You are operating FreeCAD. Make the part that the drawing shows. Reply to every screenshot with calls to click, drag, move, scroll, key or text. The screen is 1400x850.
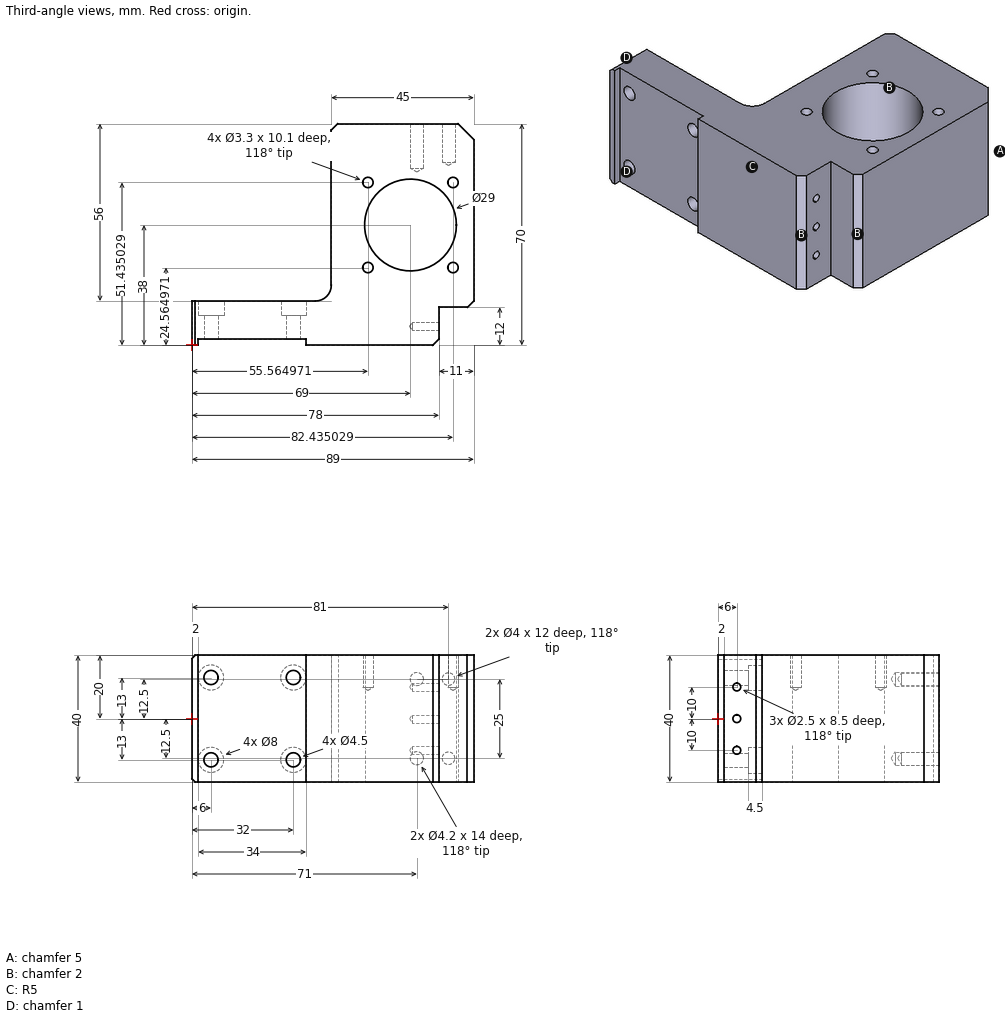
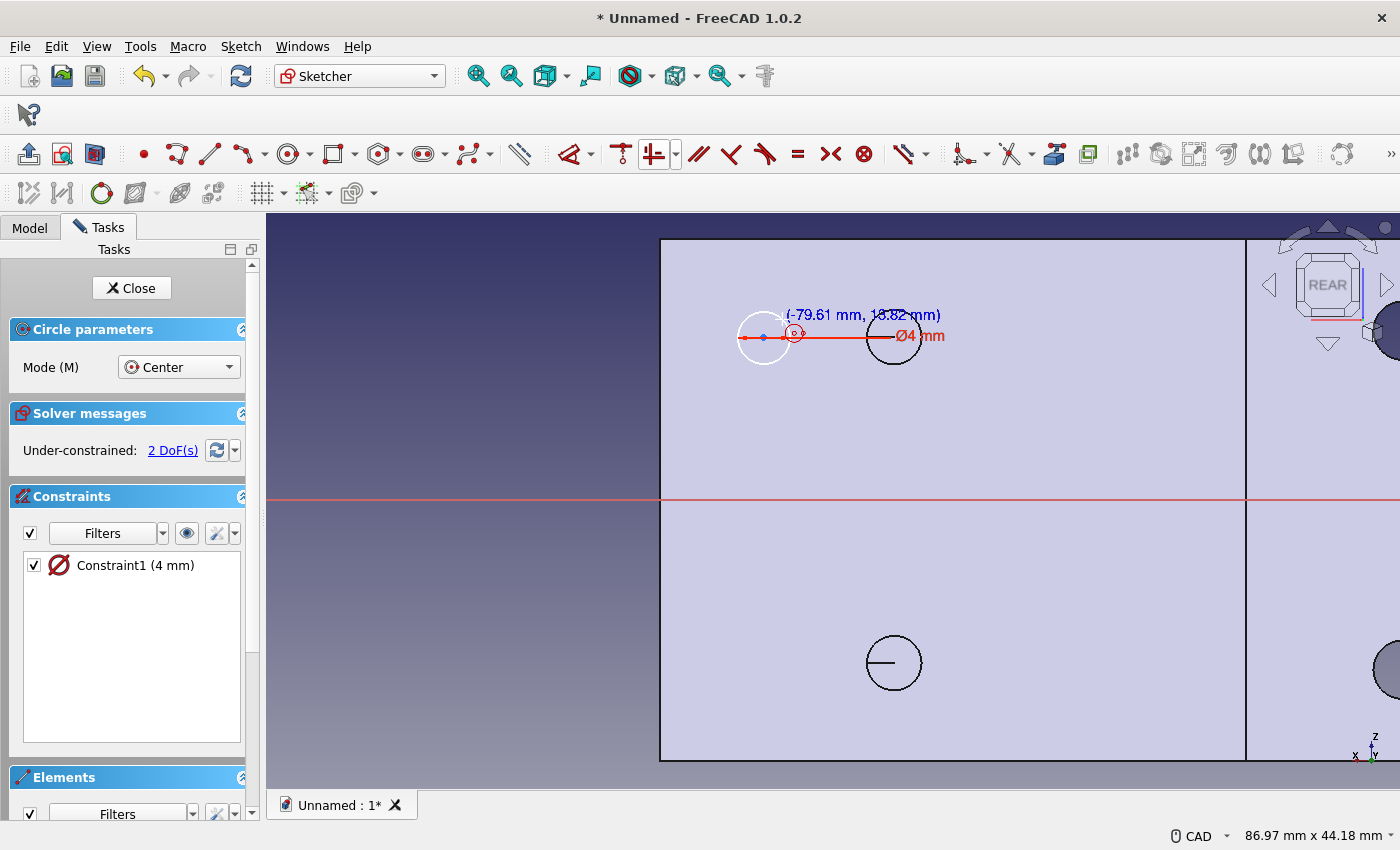
click(764, 663)
move(782, 645)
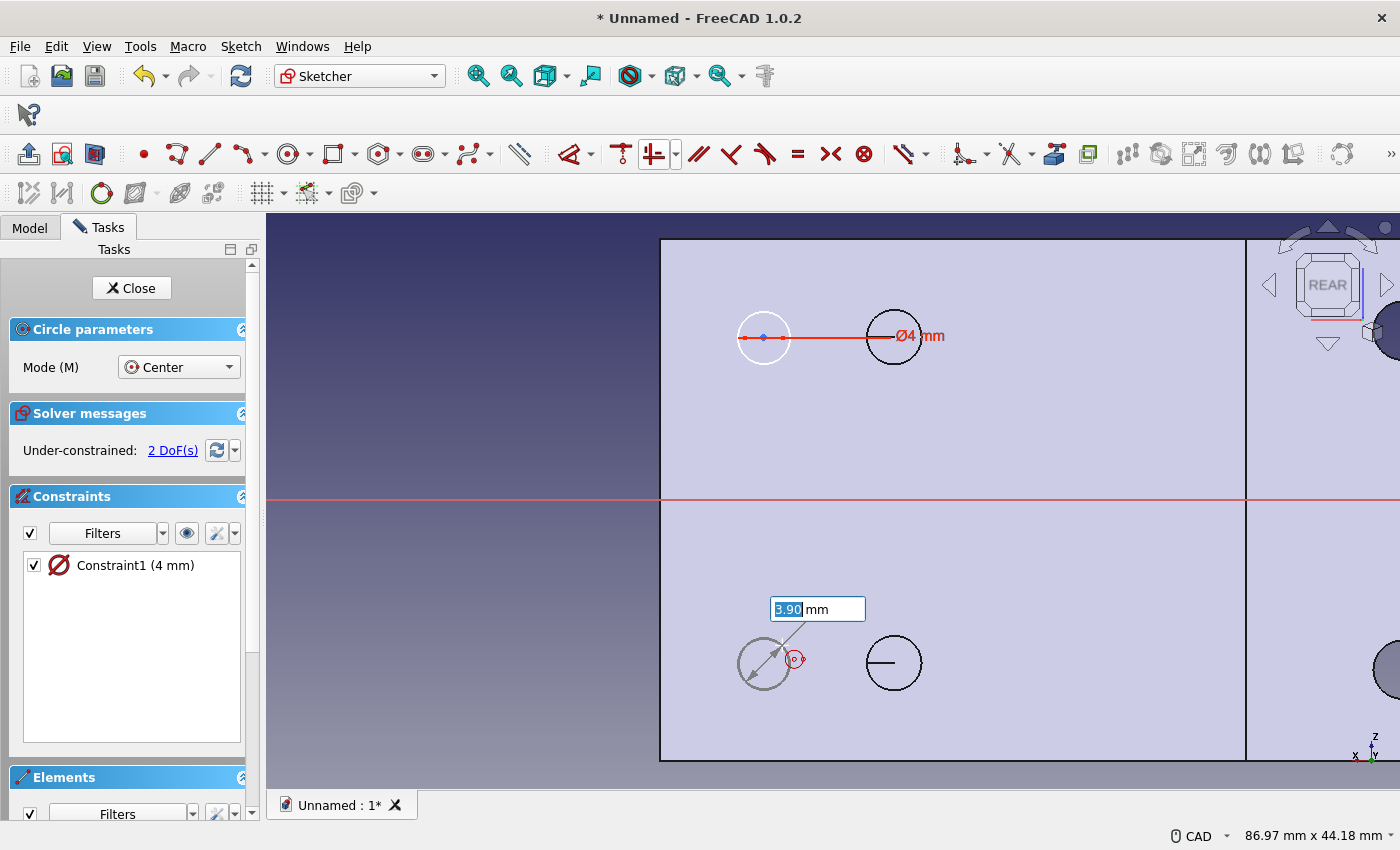
text(4)
key(Return)
key(Escape)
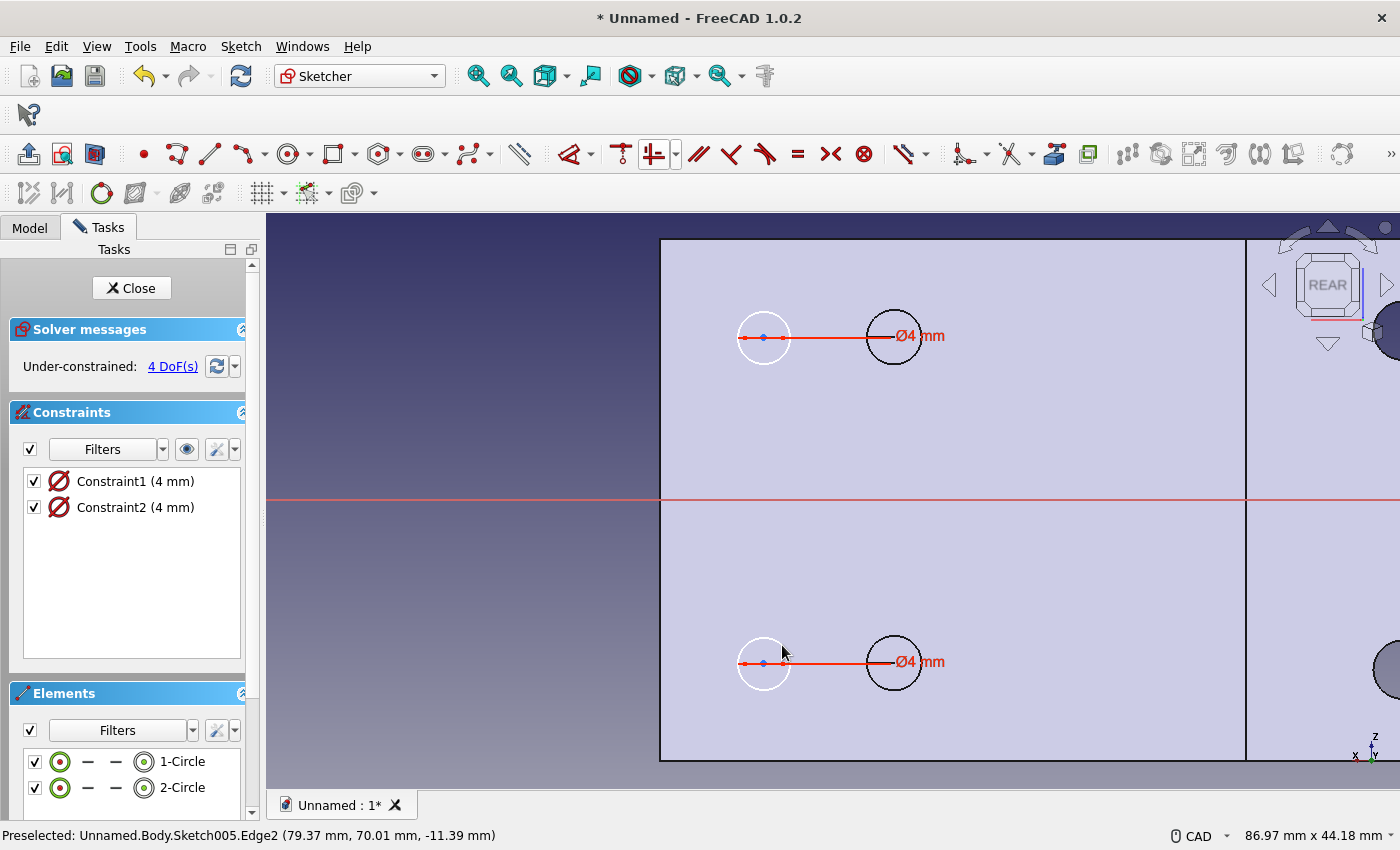
click(764, 338)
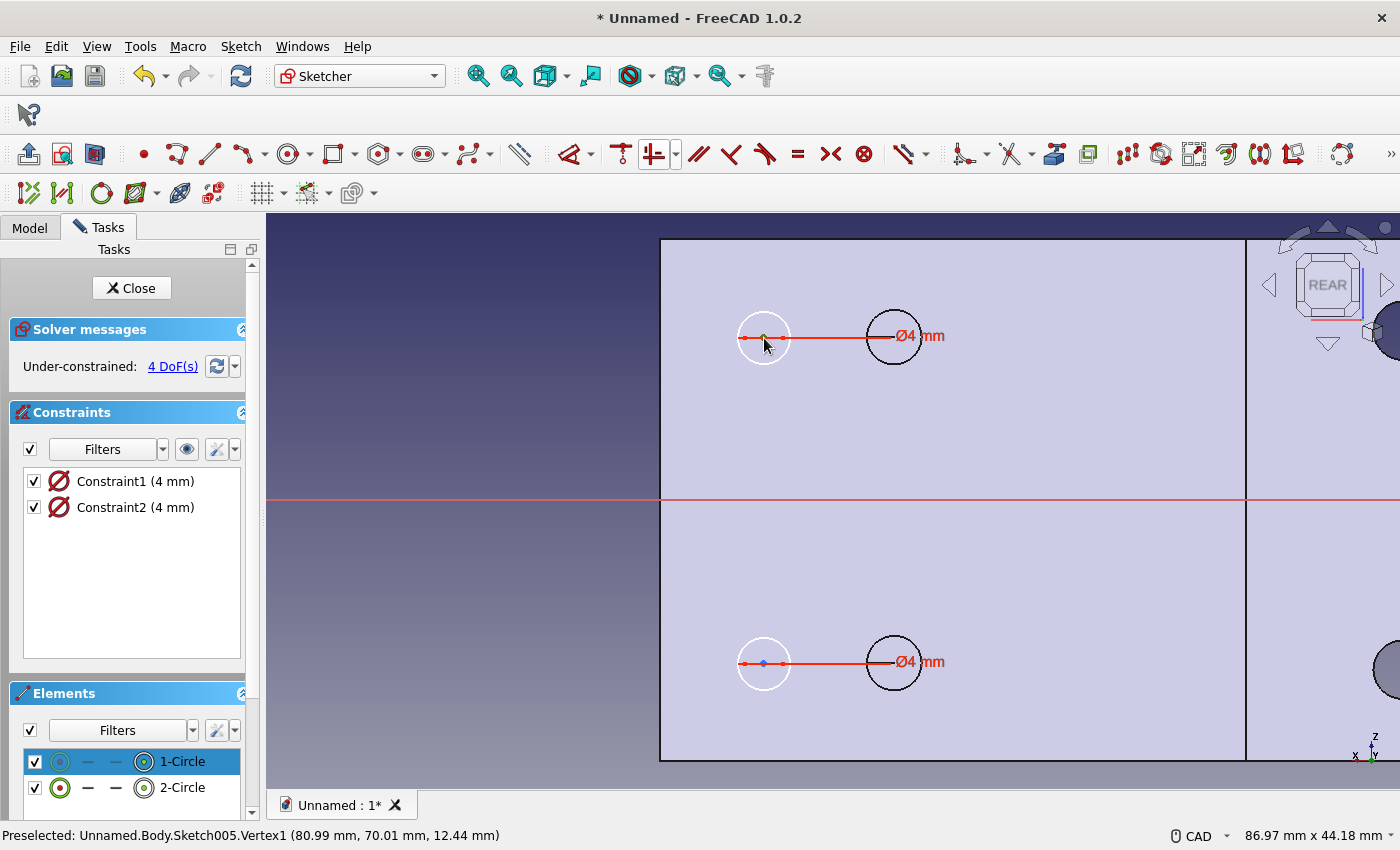
click(764, 664)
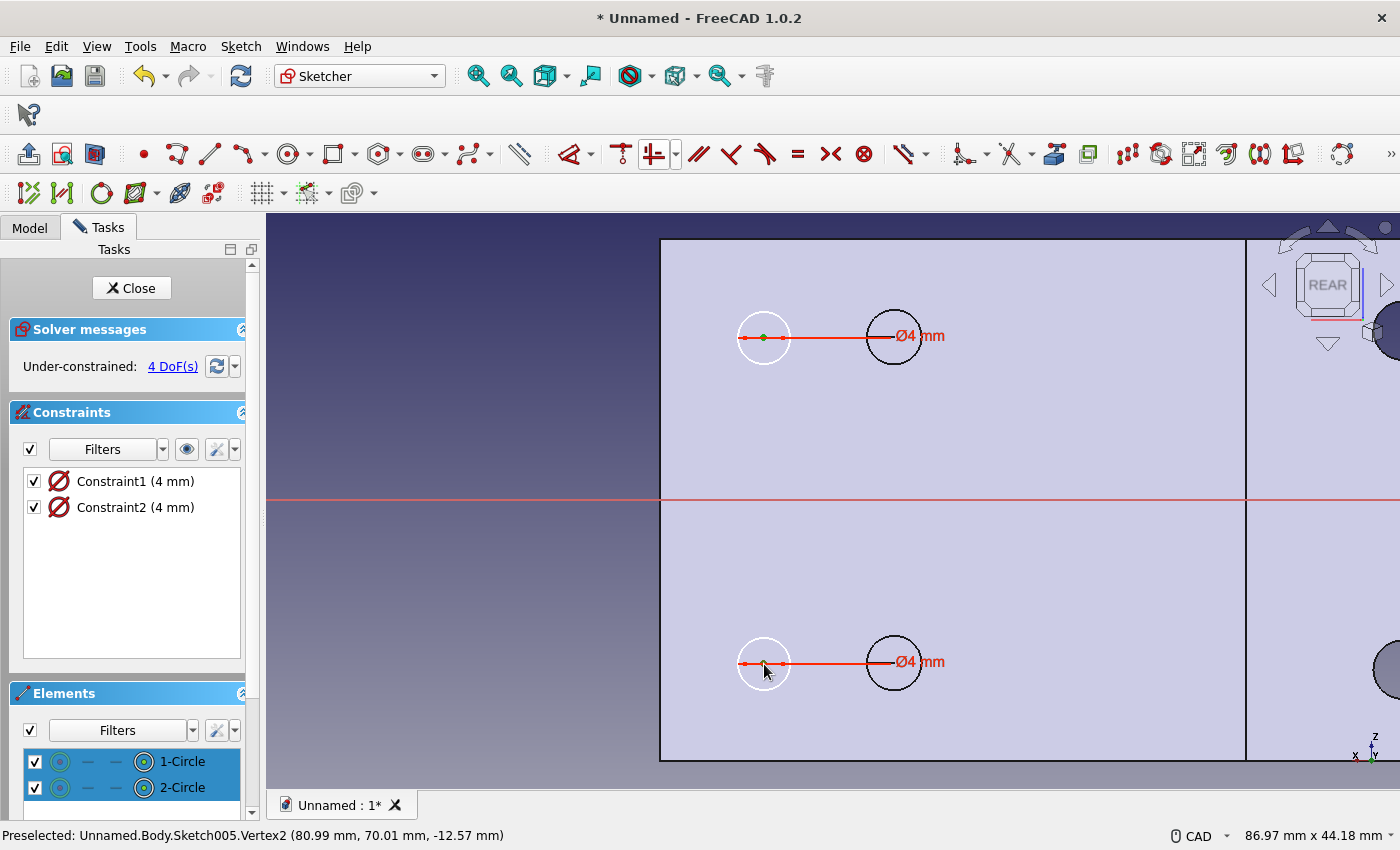
click(676, 154)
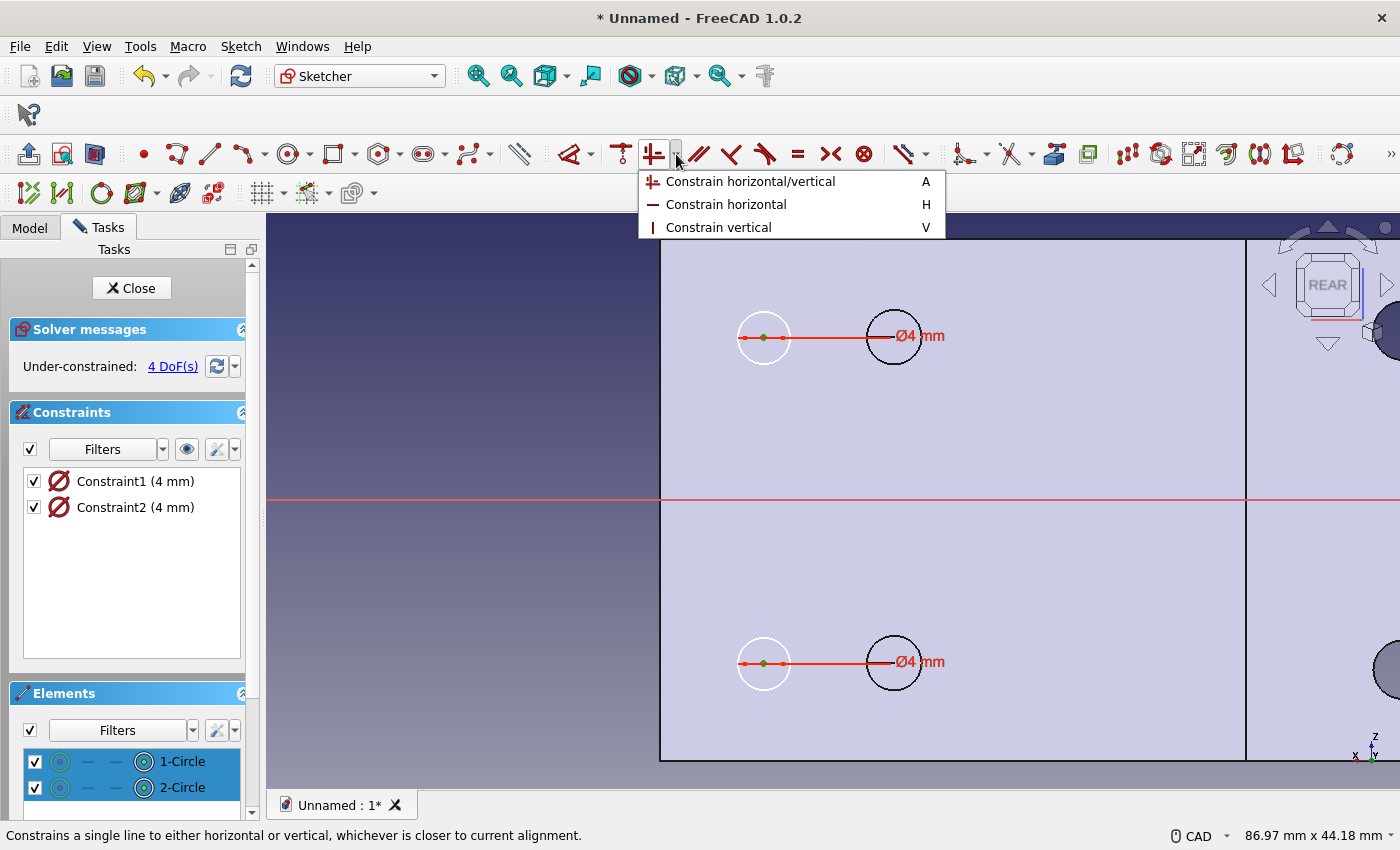
click(792, 228)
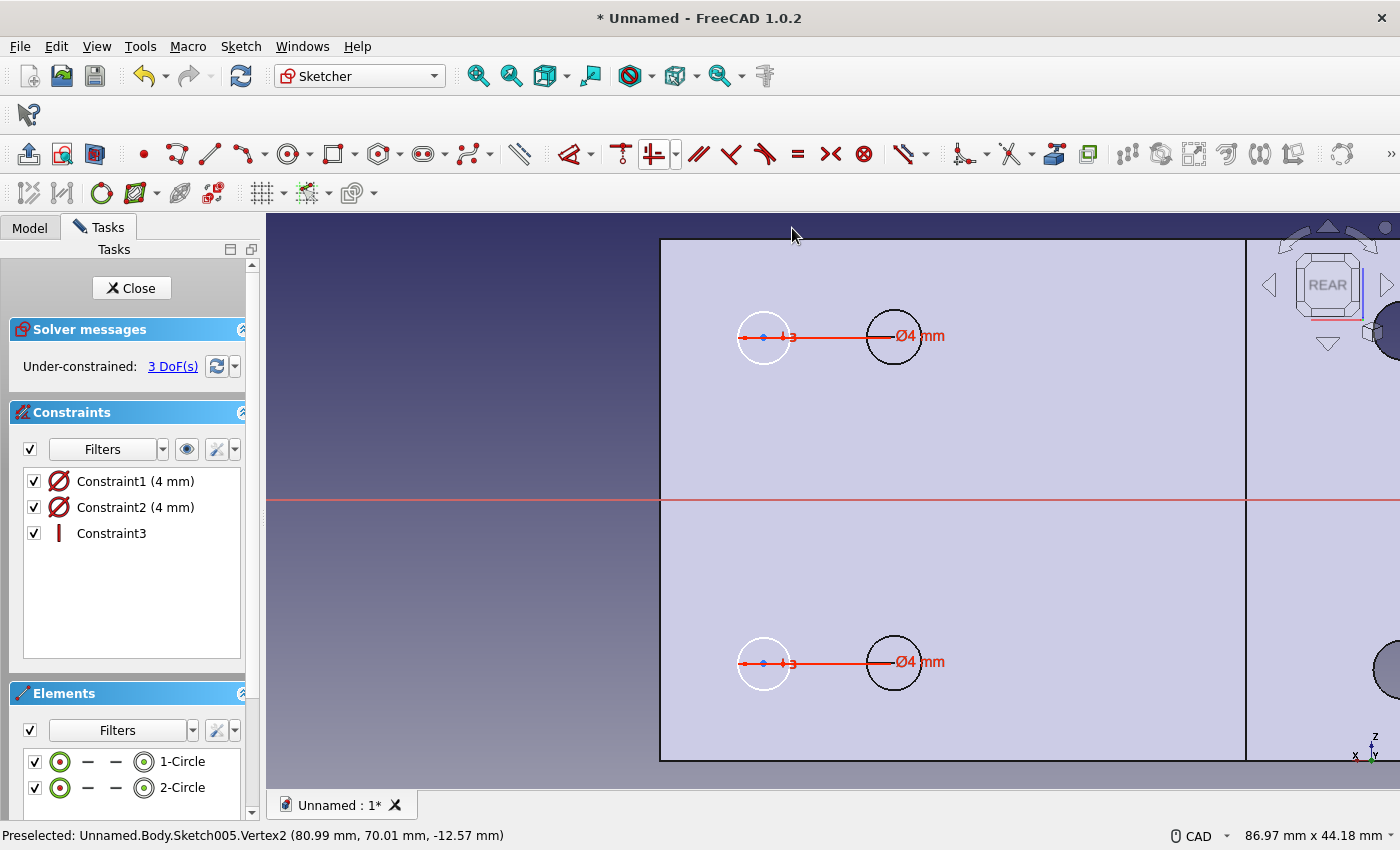
key(d)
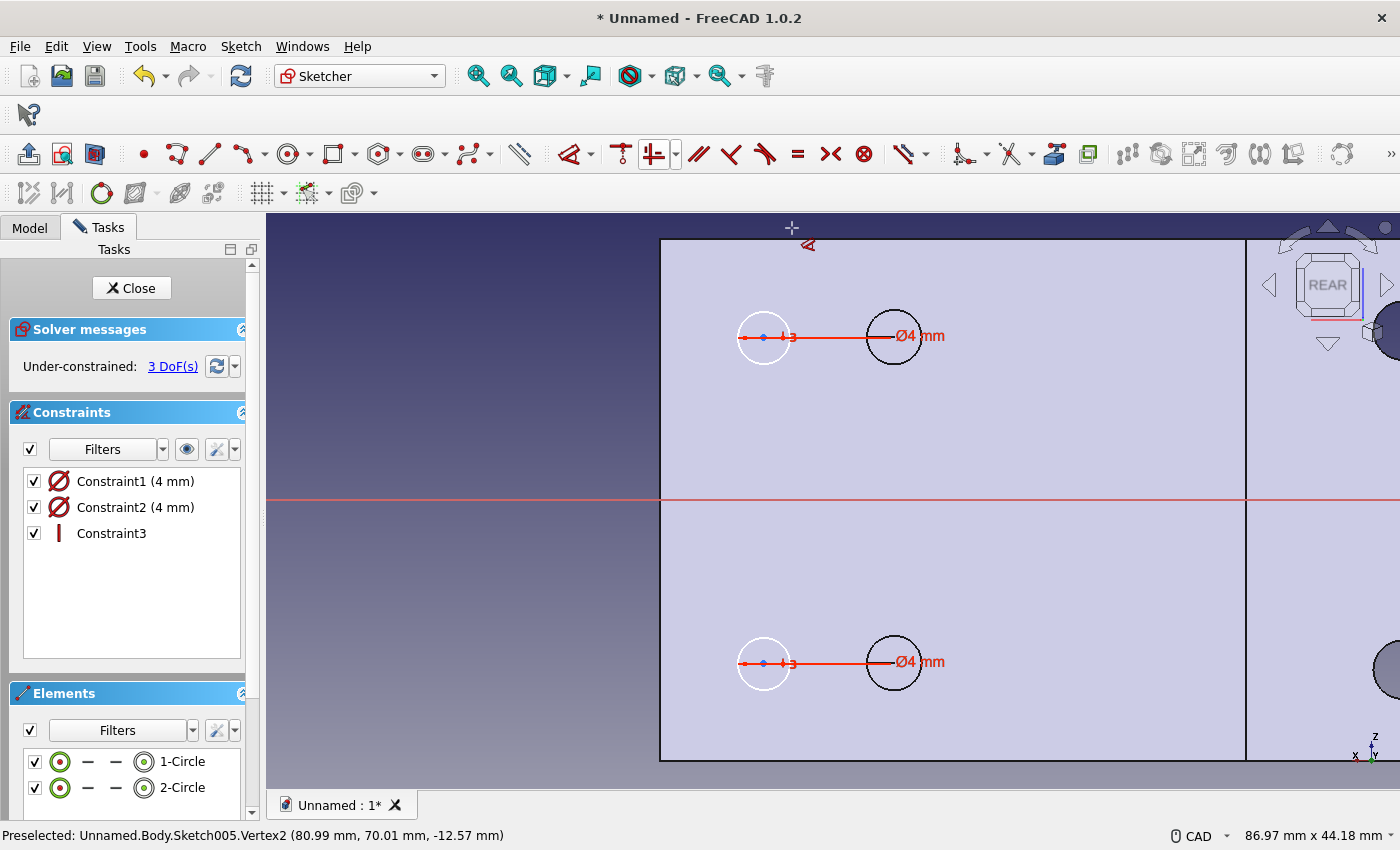
click(764, 338)
click(999, 304)